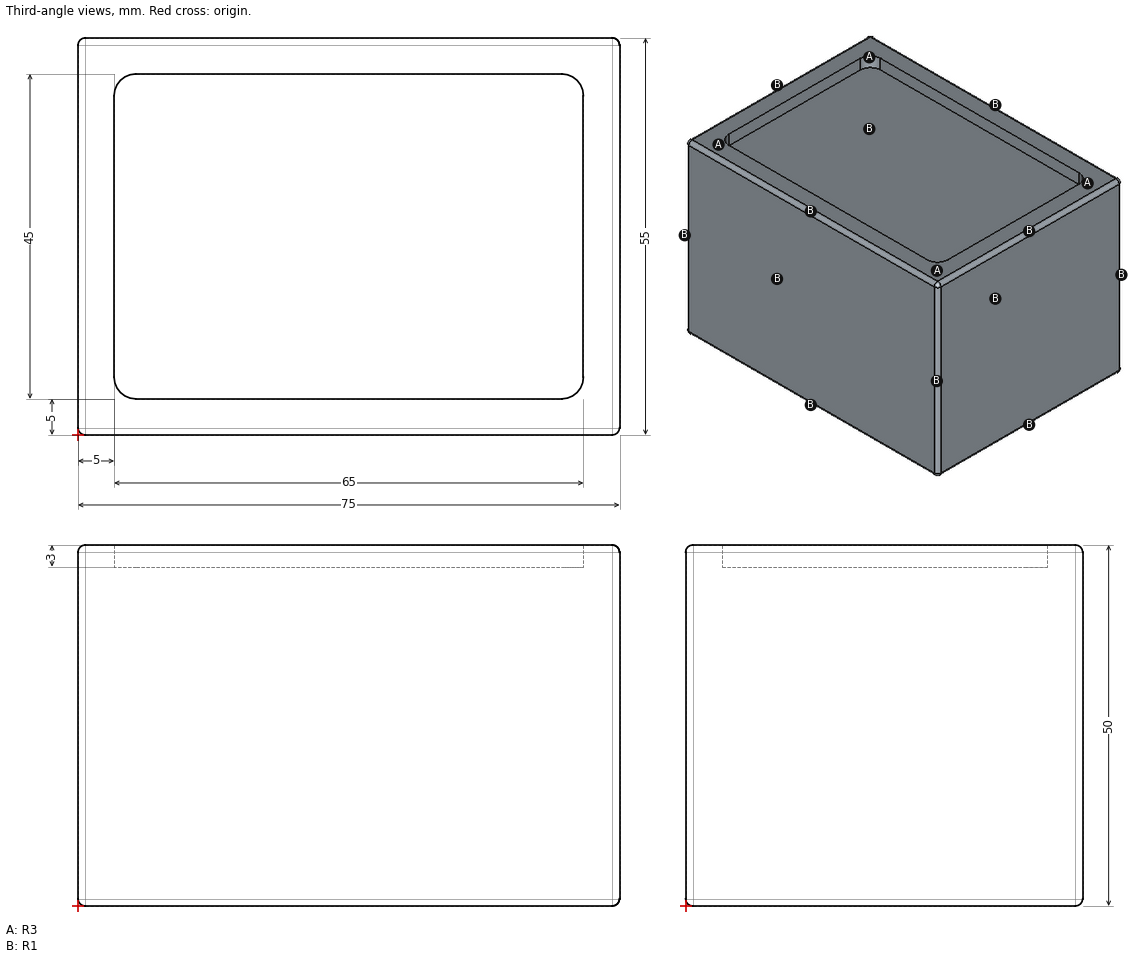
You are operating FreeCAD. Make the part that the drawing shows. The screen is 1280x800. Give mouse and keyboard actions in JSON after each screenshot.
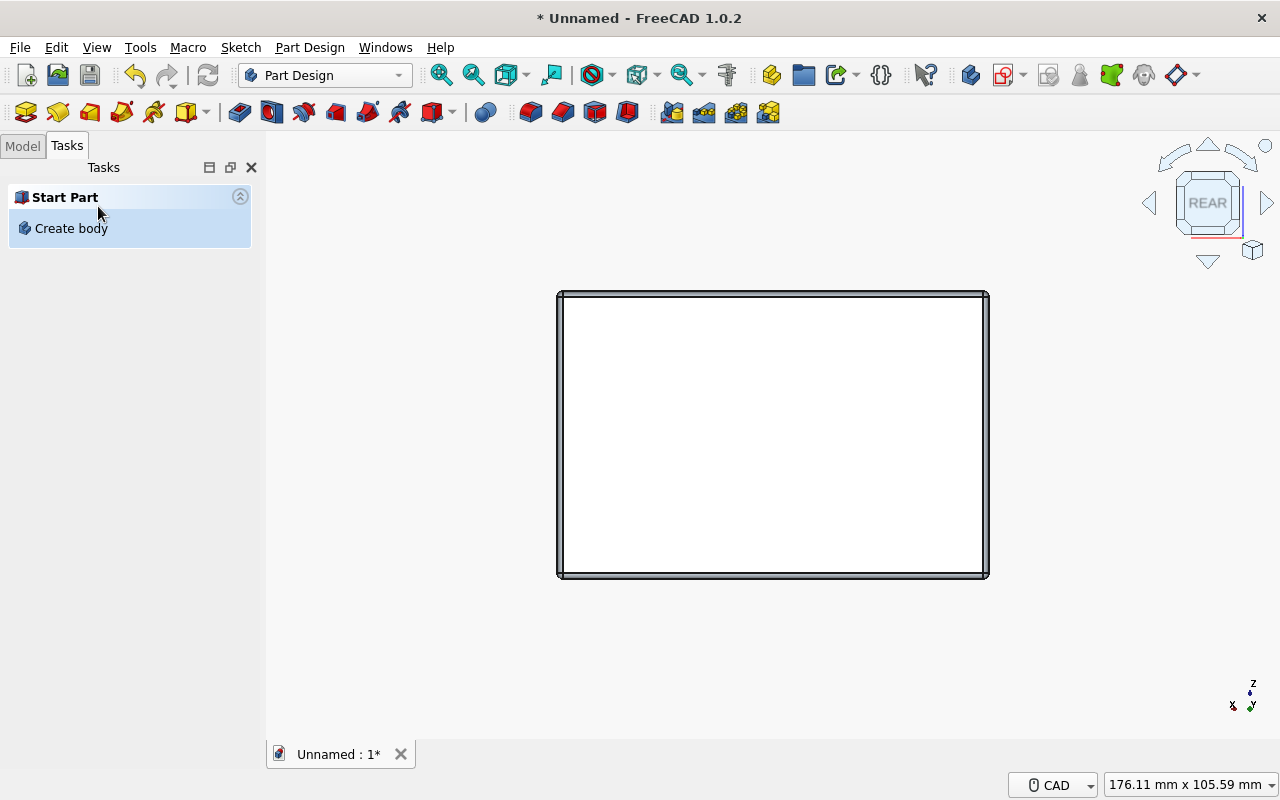
{"action": "key", "text": "0"}